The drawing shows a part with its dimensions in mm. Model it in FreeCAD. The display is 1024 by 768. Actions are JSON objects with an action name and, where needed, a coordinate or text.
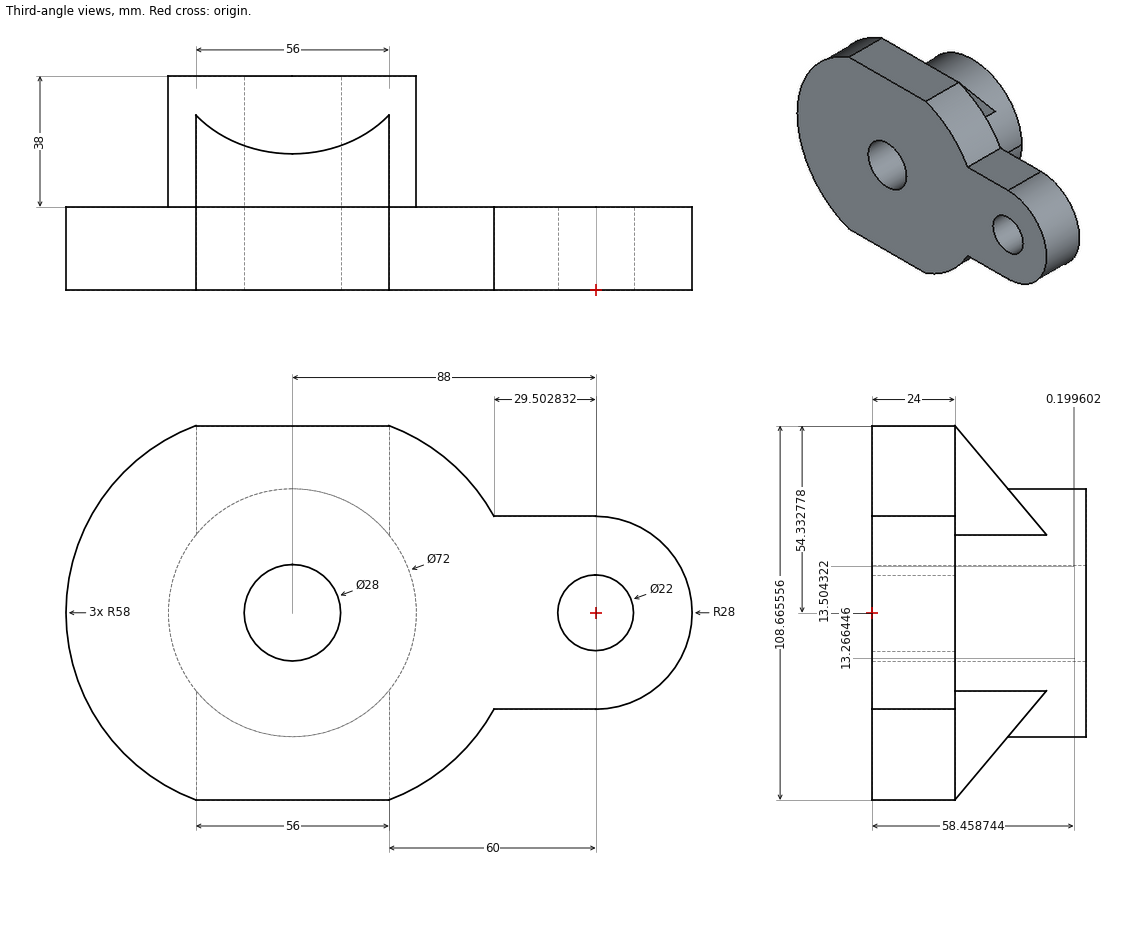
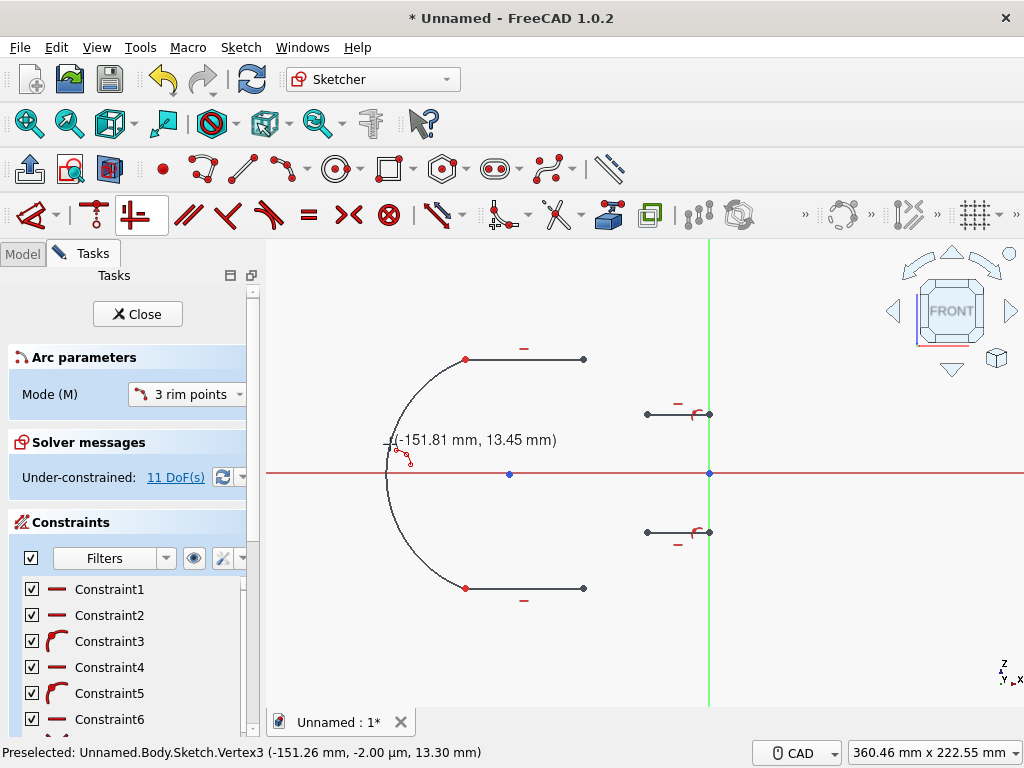
{"action": "left_click", "coordinate": [583, 360]}
{"action": "left_click", "coordinate": [647, 415]}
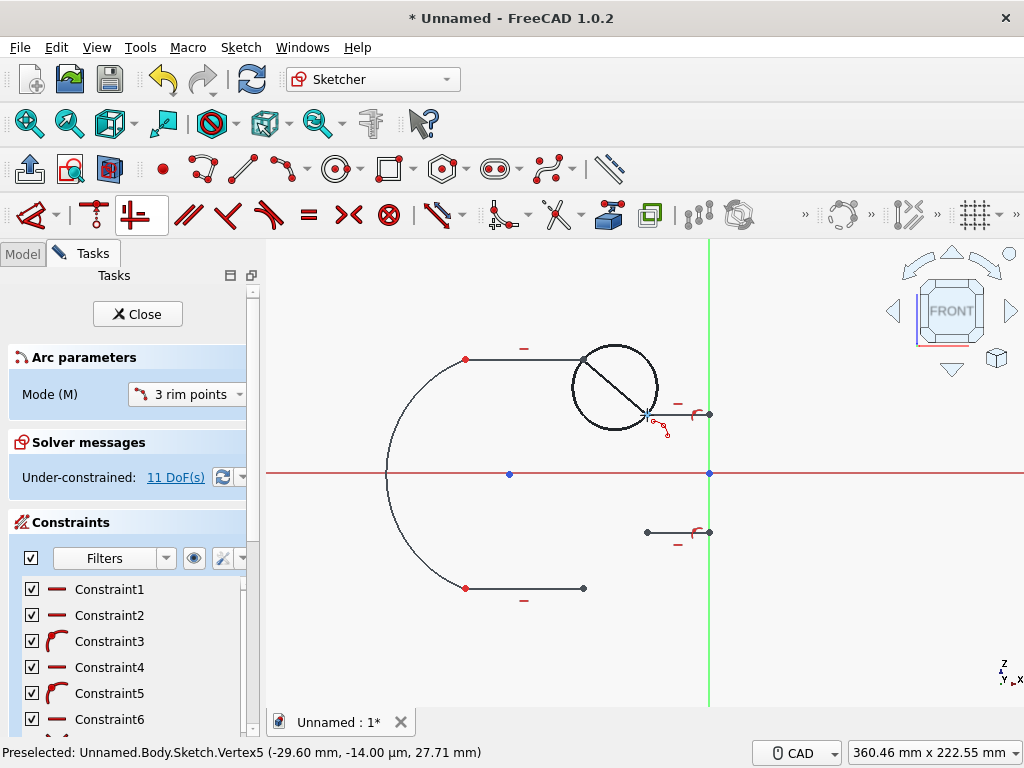
{"action": "scroll", "coordinate": [620, 381], "scroll_direction": "up", "scroll_amount": 4}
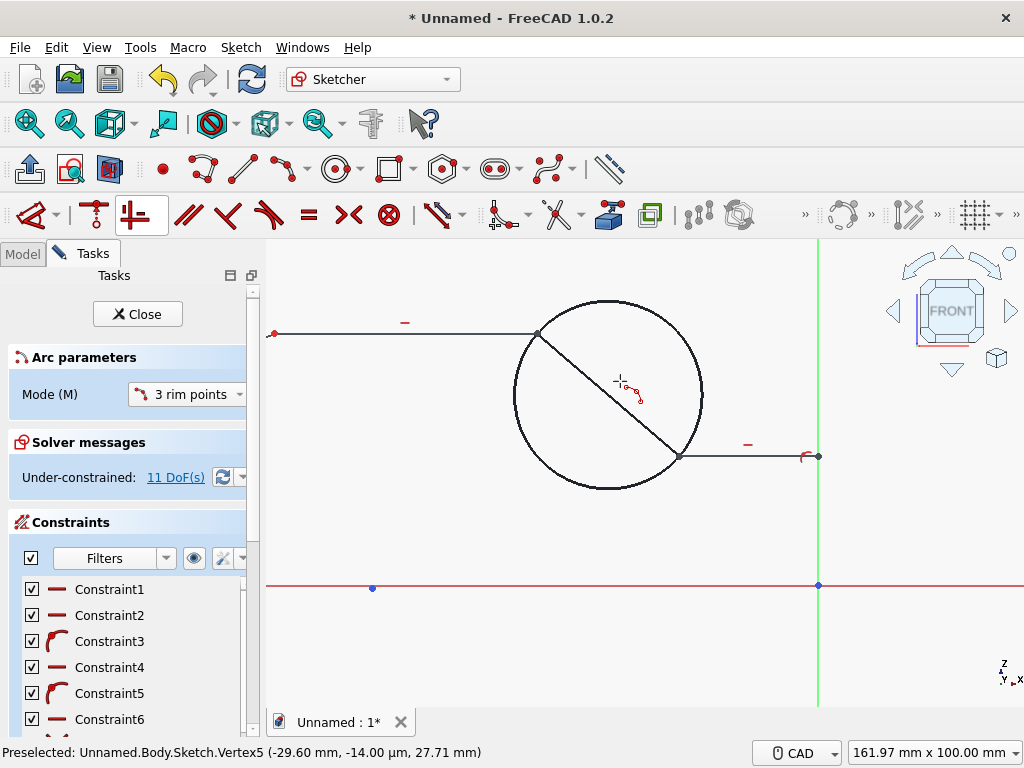
{"action": "left_click", "coordinate": [620, 381]}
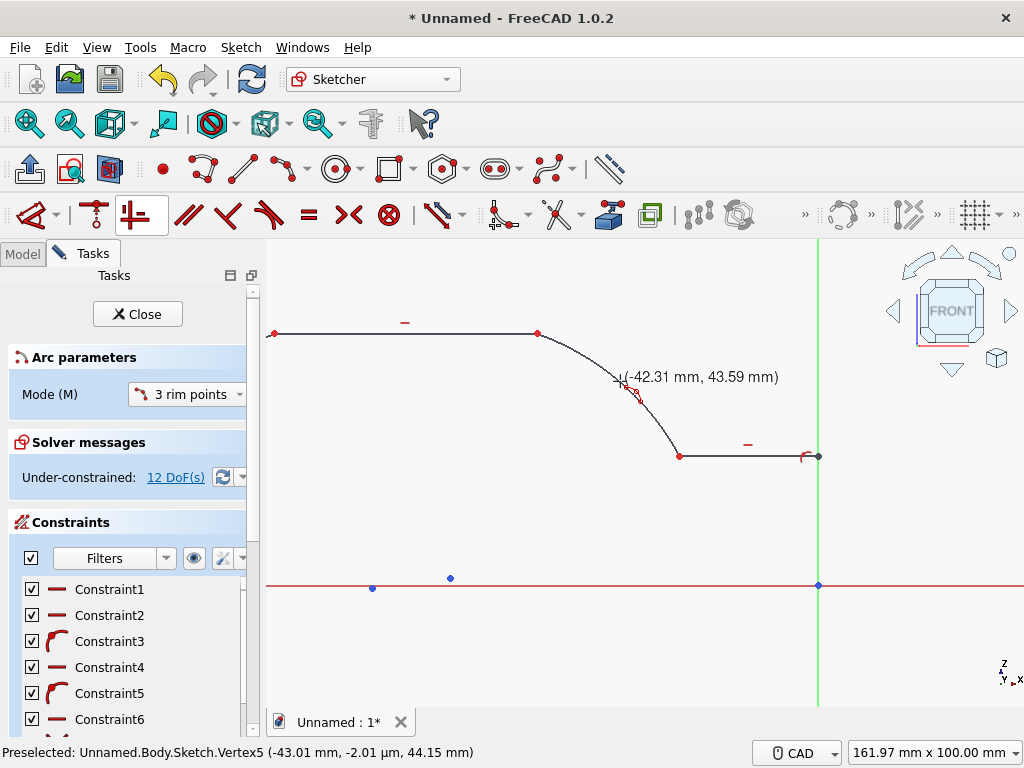
{"action": "left_click", "coordinate": [818, 456]}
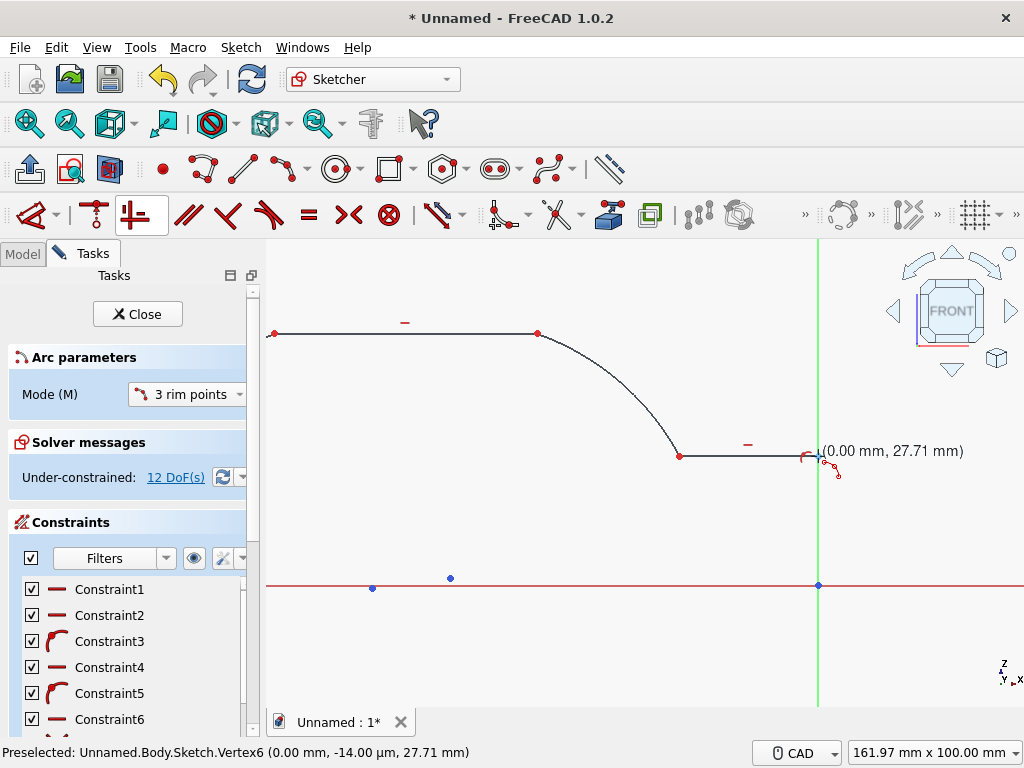
{"action": "scroll", "coordinate": [619, 381], "scroll_direction": "down", "scroll_amount": 4}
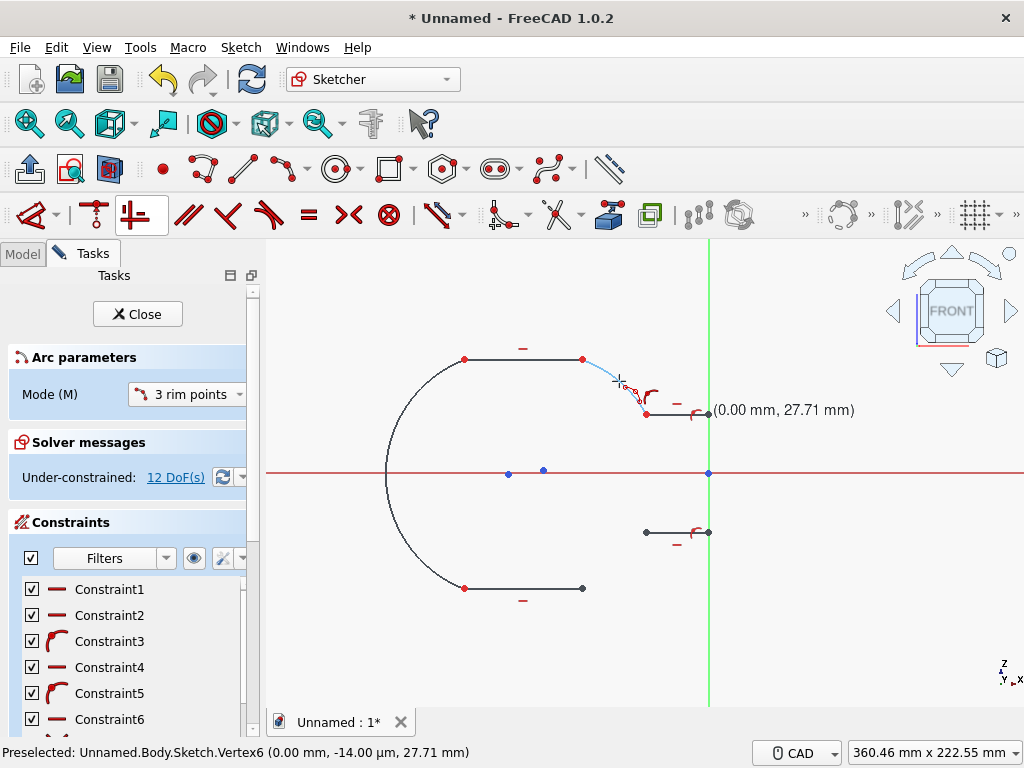
{"action": "left_click", "coordinate": [709, 533]}
{"action": "left_click", "coordinate": [765, 491]}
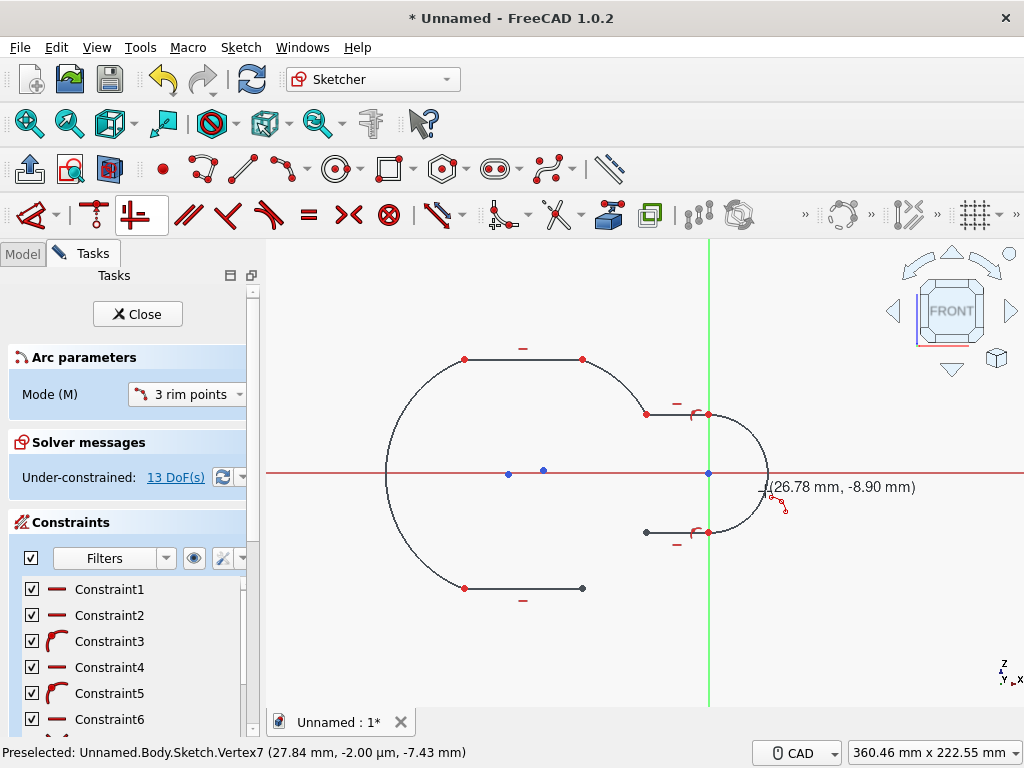
{"action": "left_click", "coordinate": [646, 533]}
{"action": "left_click", "coordinate": [582, 589]}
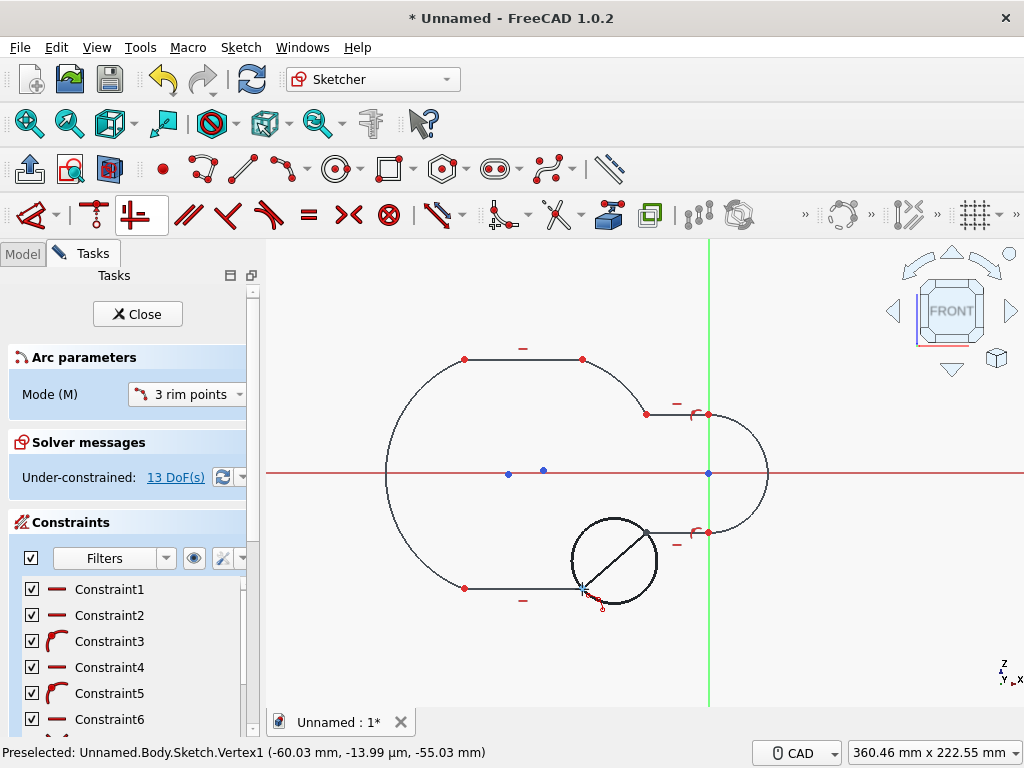
{"action": "scroll", "coordinate": [620, 566], "scroll_direction": "up", "scroll_amount": 4}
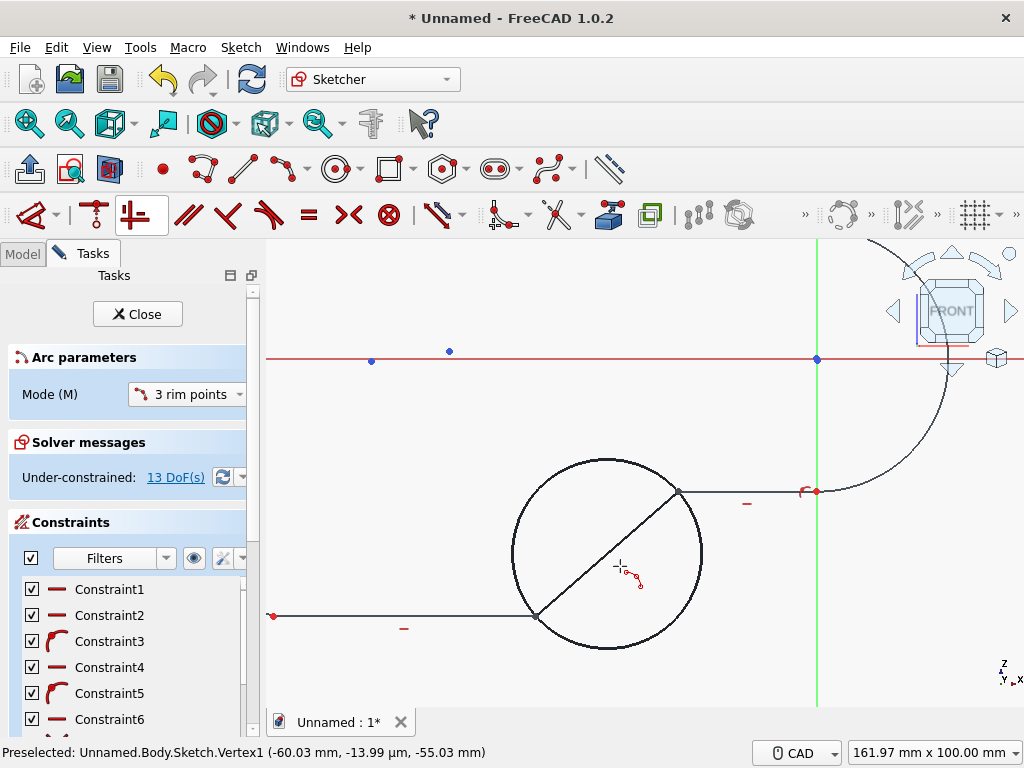
{"action": "left_click", "coordinate": [618, 564]}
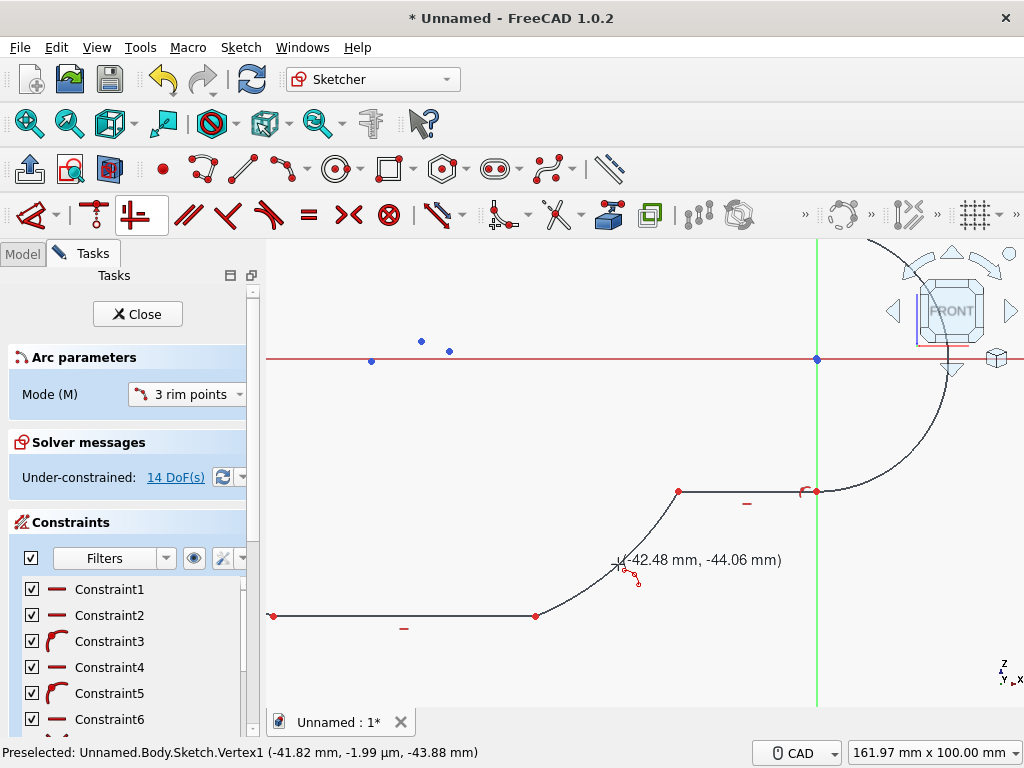
{"action": "left_click", "coordinate": [336, 170]}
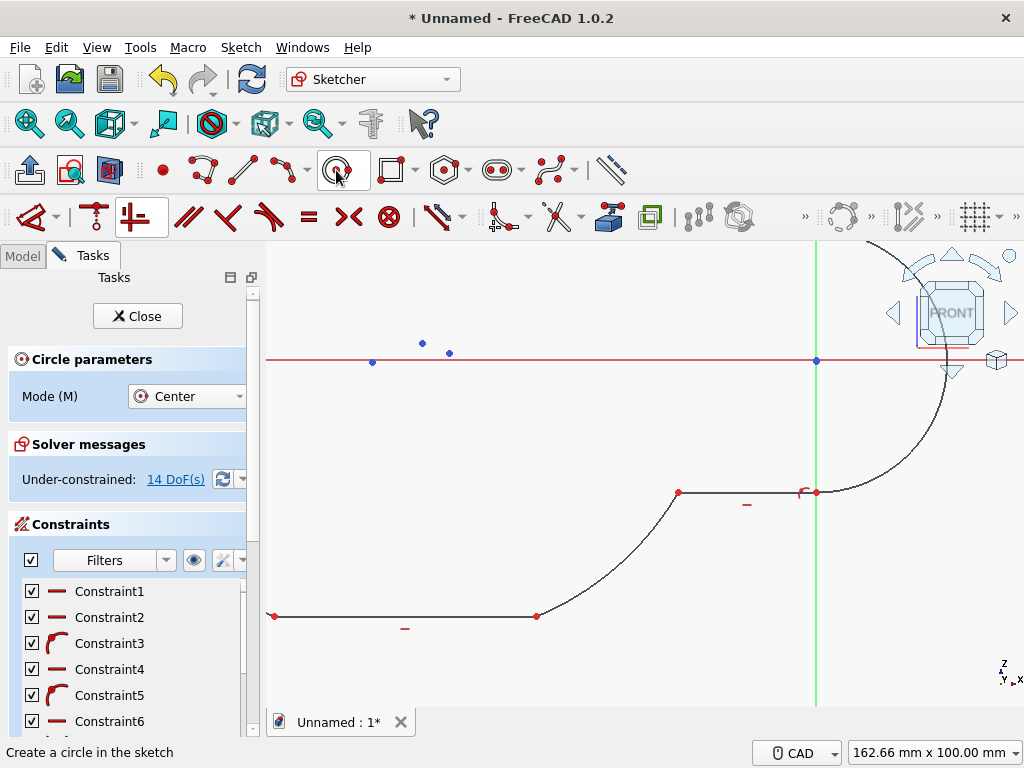
{"action": "left_click", "coordinate": [816, 360]}
{"action": "mouse_move", "coordinate": [852, 324]}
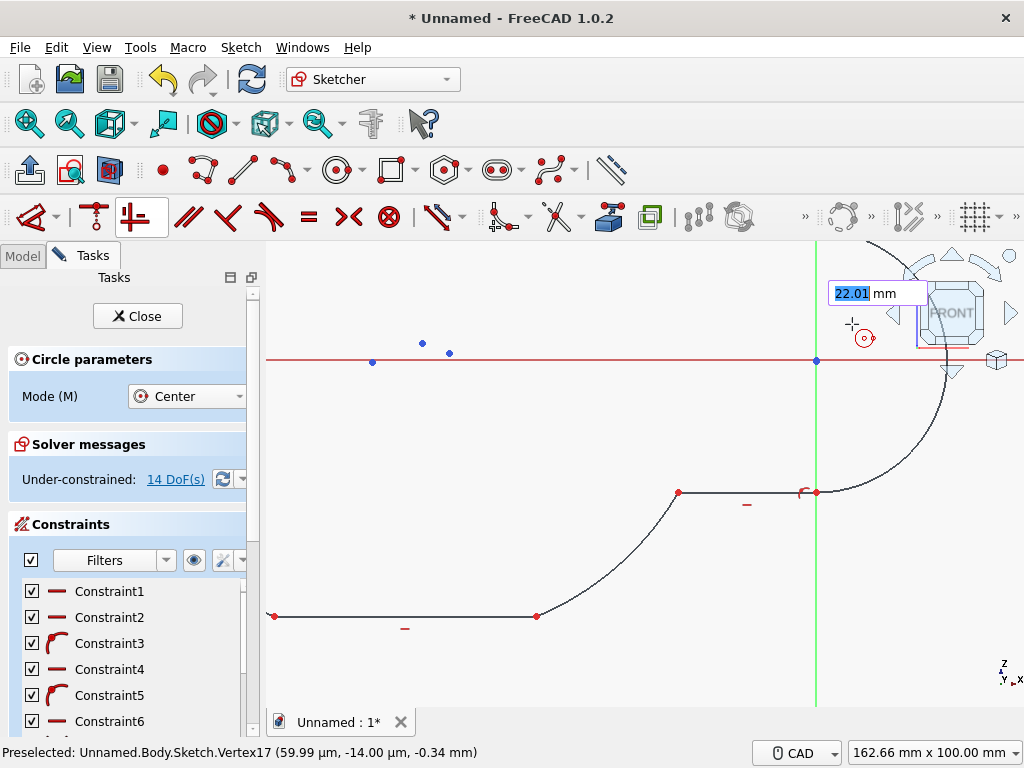
{"action": "type", "text": "22"}
{"action": "key", "text": "Return"}
{"action": "key", "text": "Escape"}